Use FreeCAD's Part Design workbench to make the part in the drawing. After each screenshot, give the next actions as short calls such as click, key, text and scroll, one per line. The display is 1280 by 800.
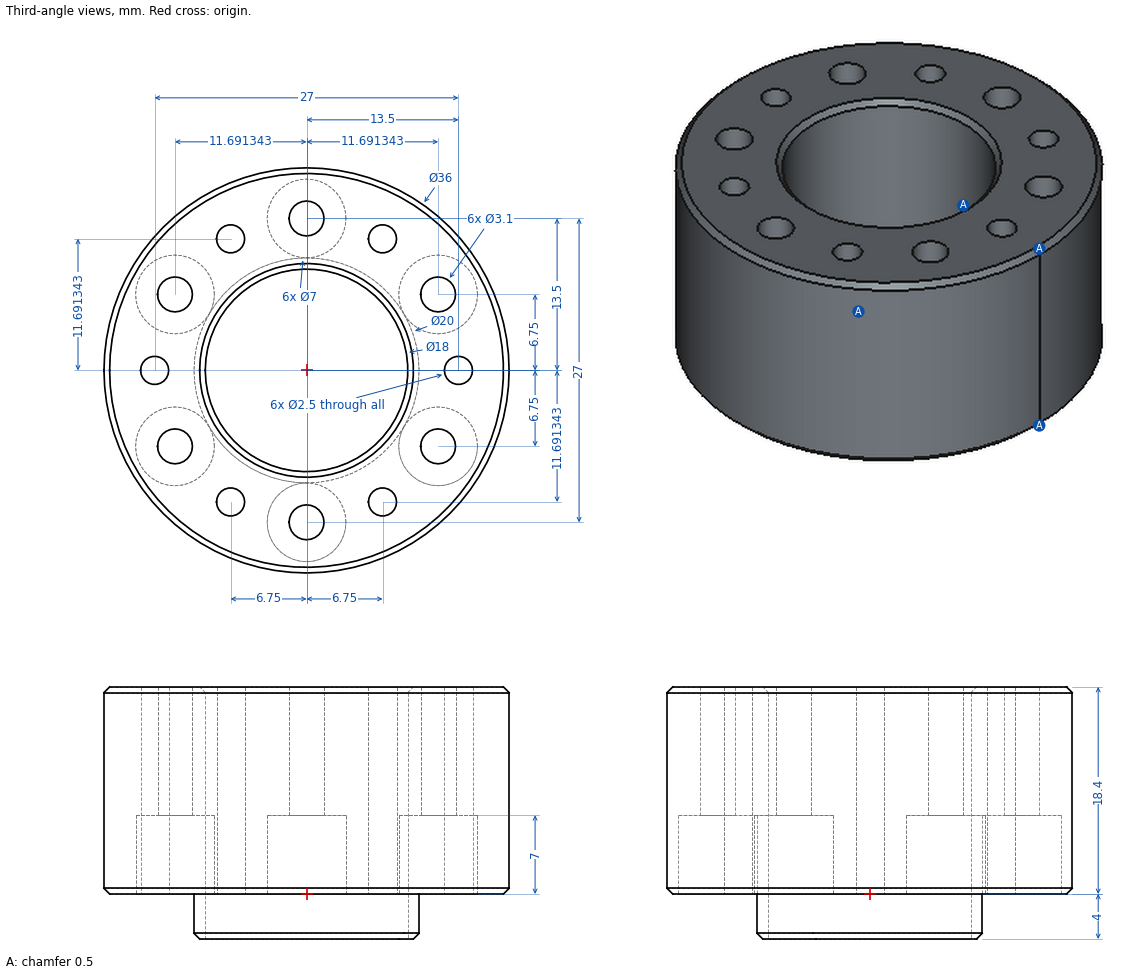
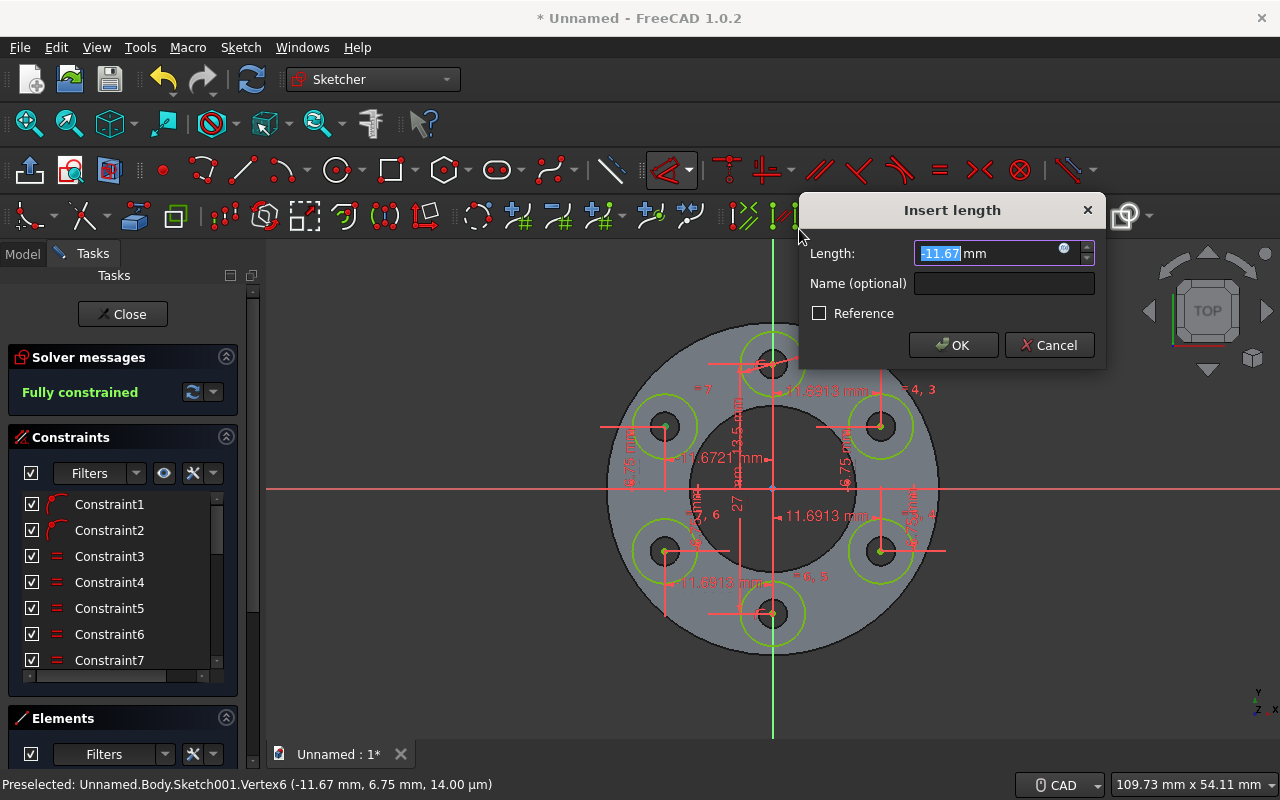
text(-11.691343)
key(Return)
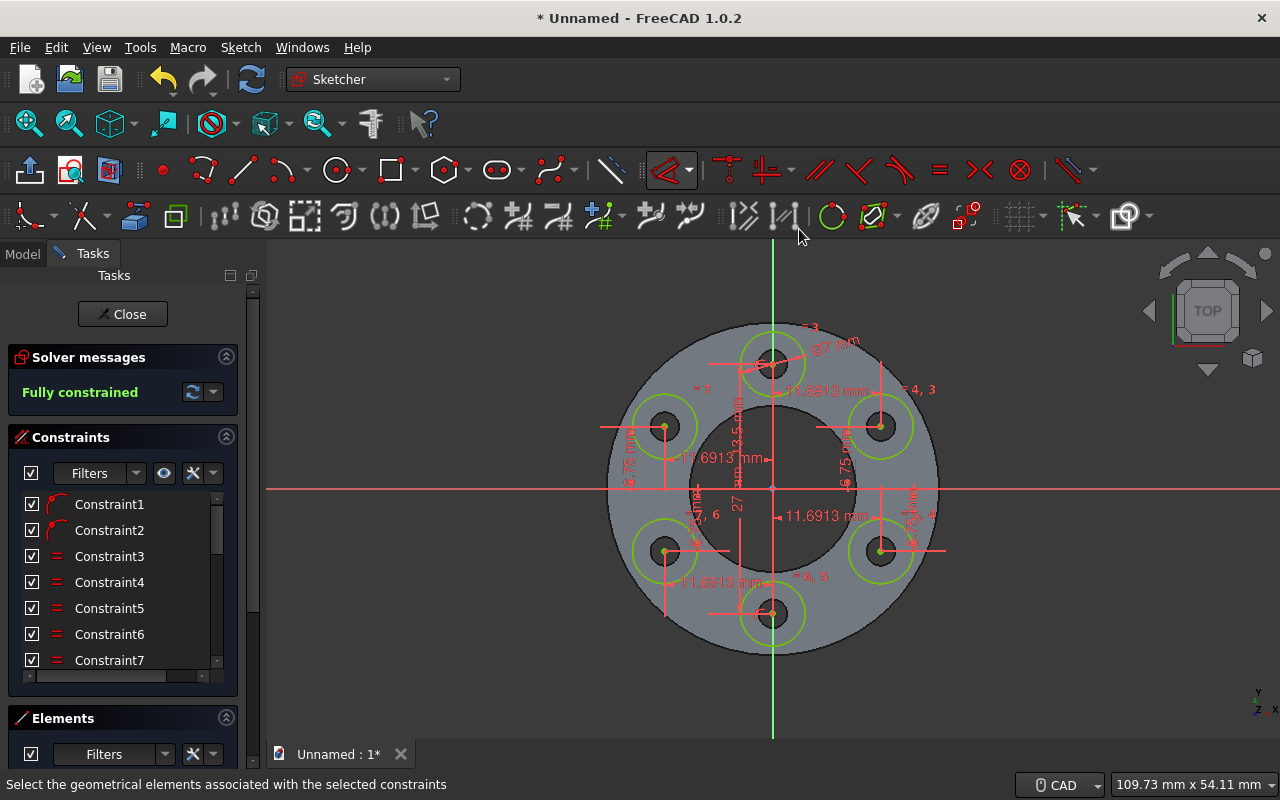
click(123, 314)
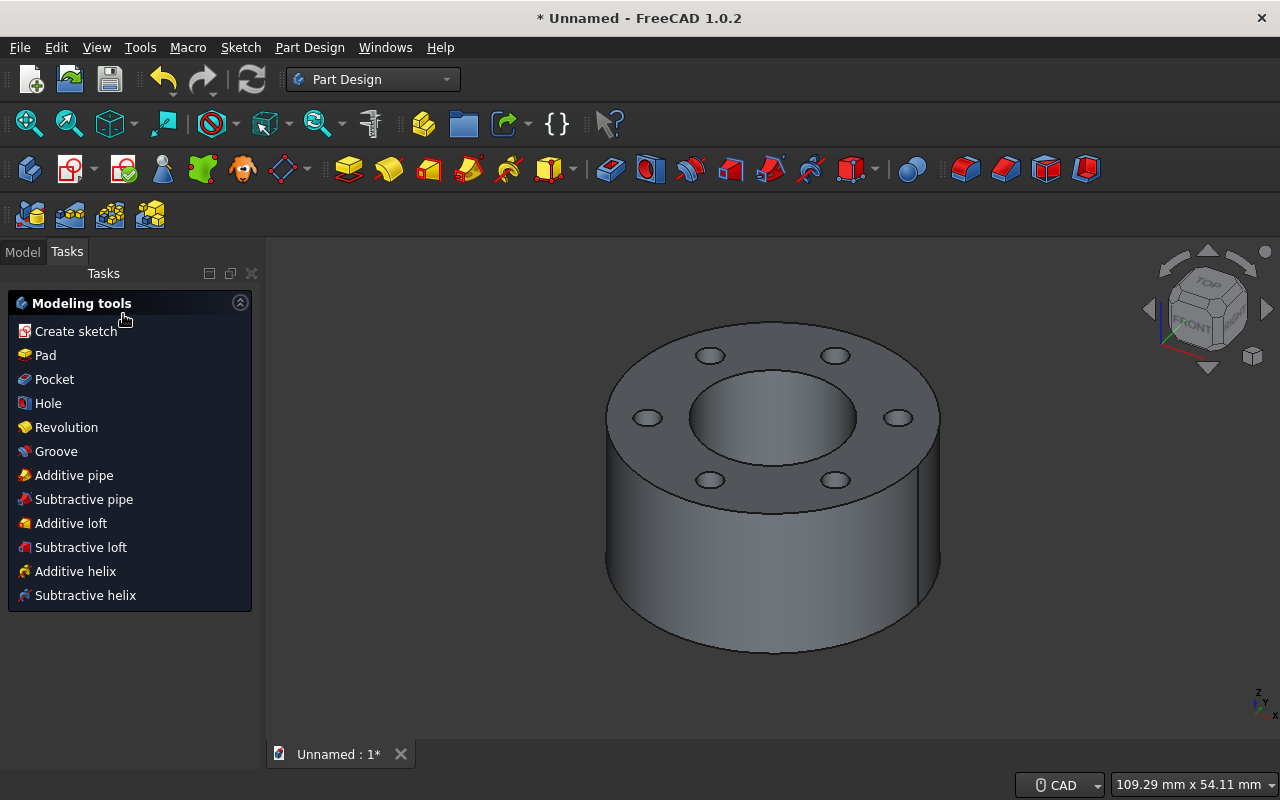
click(612, 170)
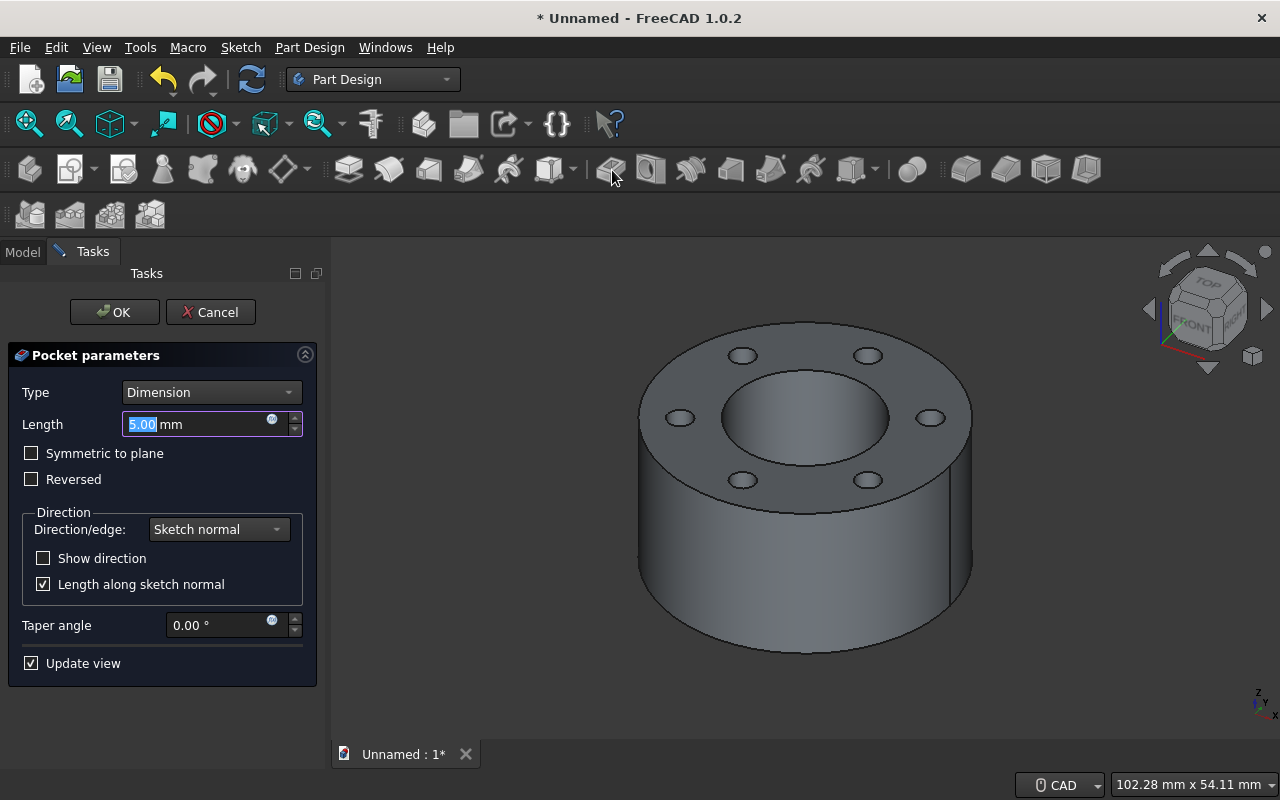
text(7)
key(Tab)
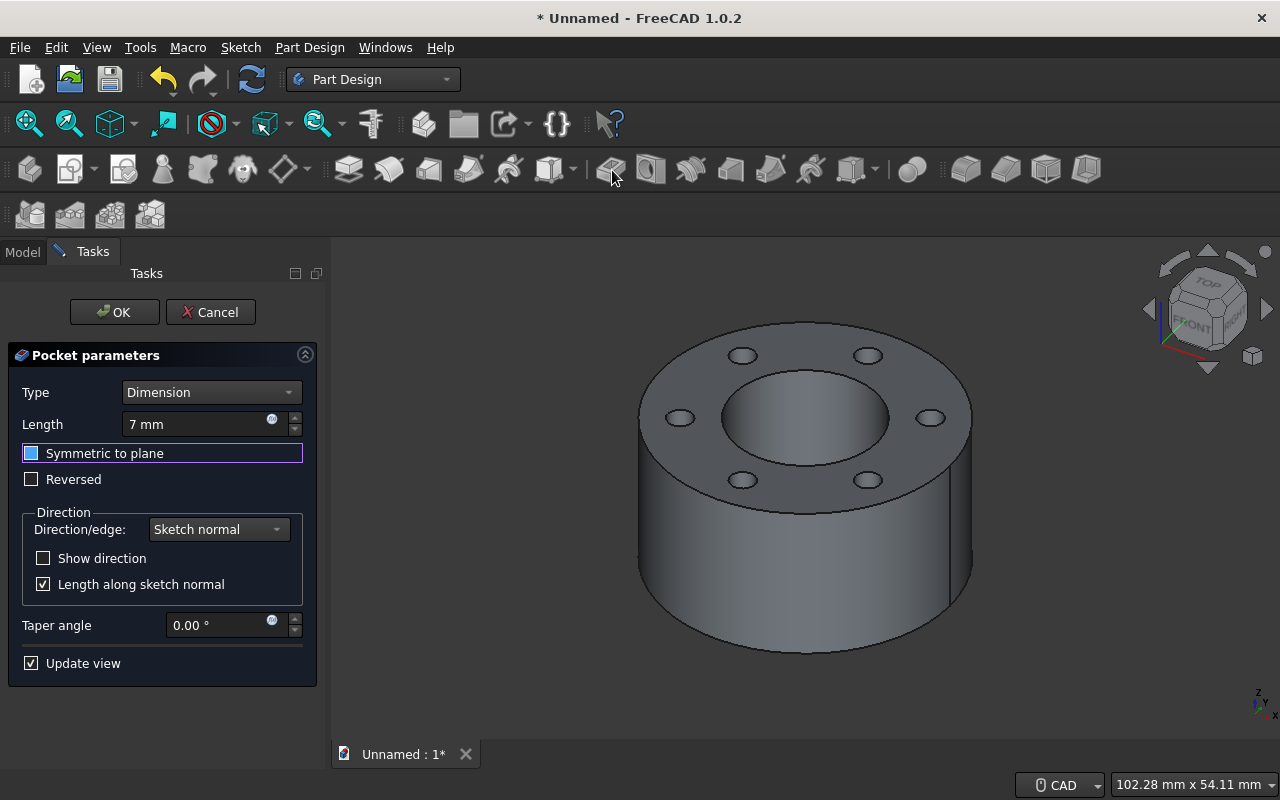
click(30, 479)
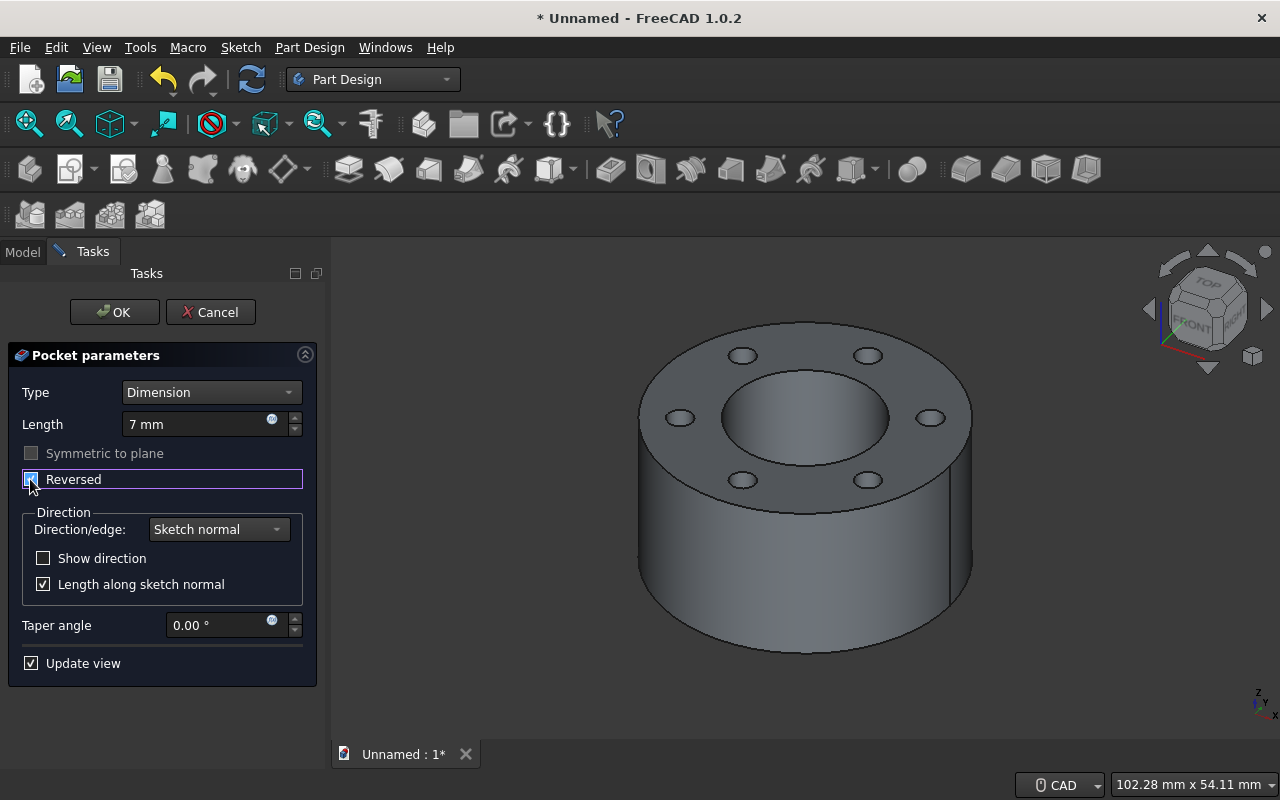
click(115, 312)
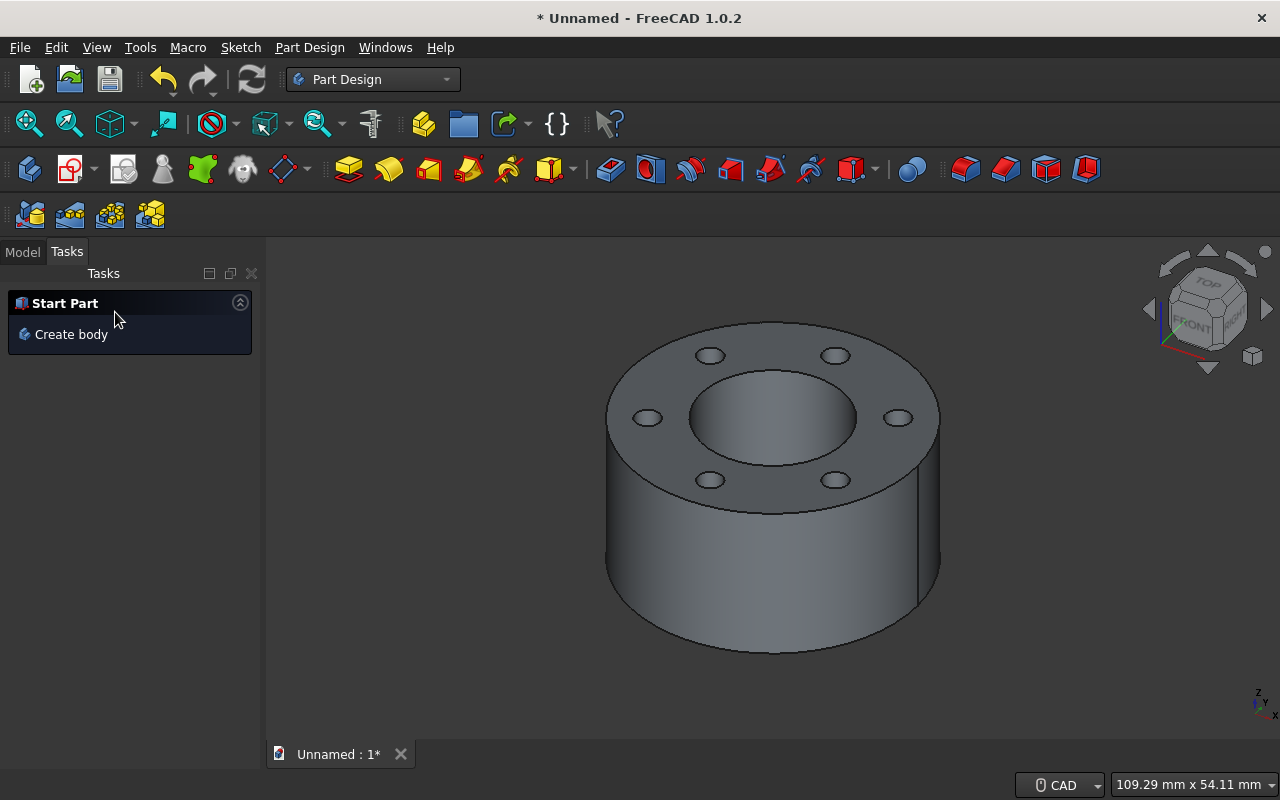
click(23, 251)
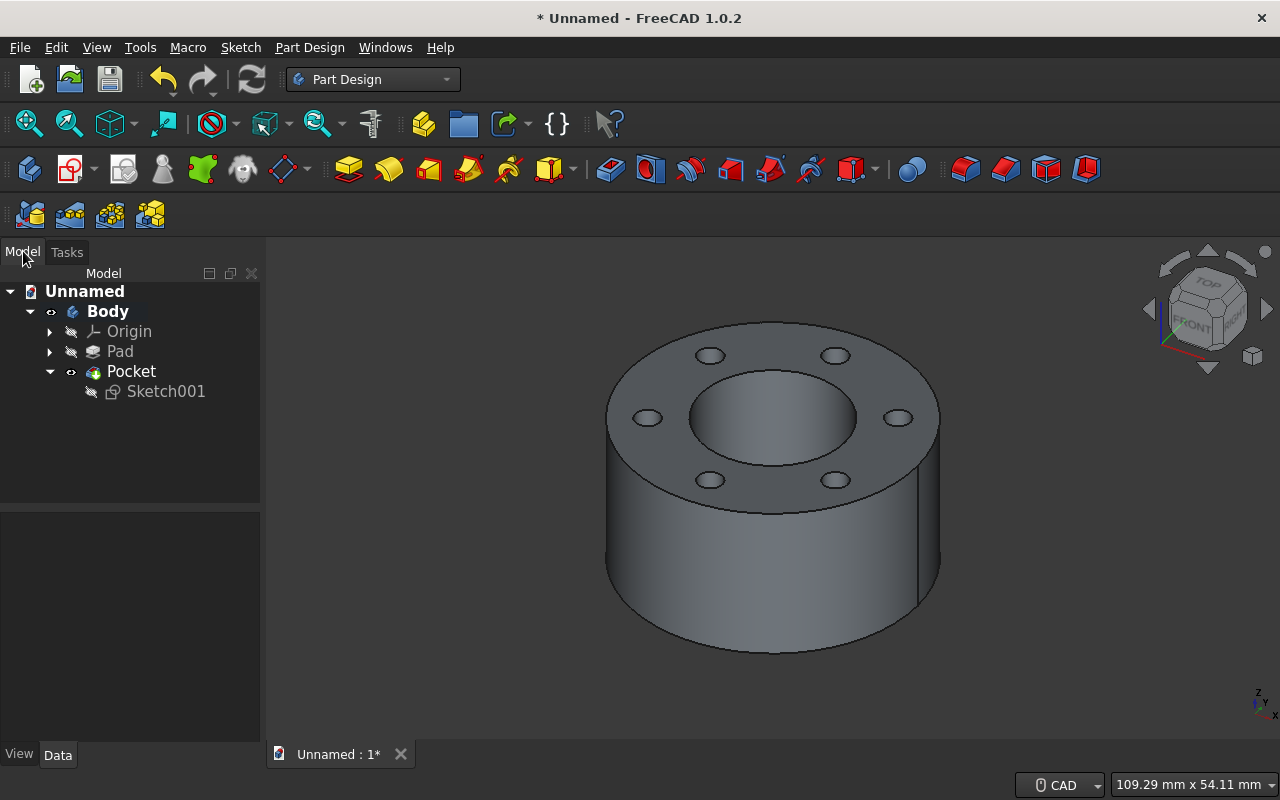
click(50, 332)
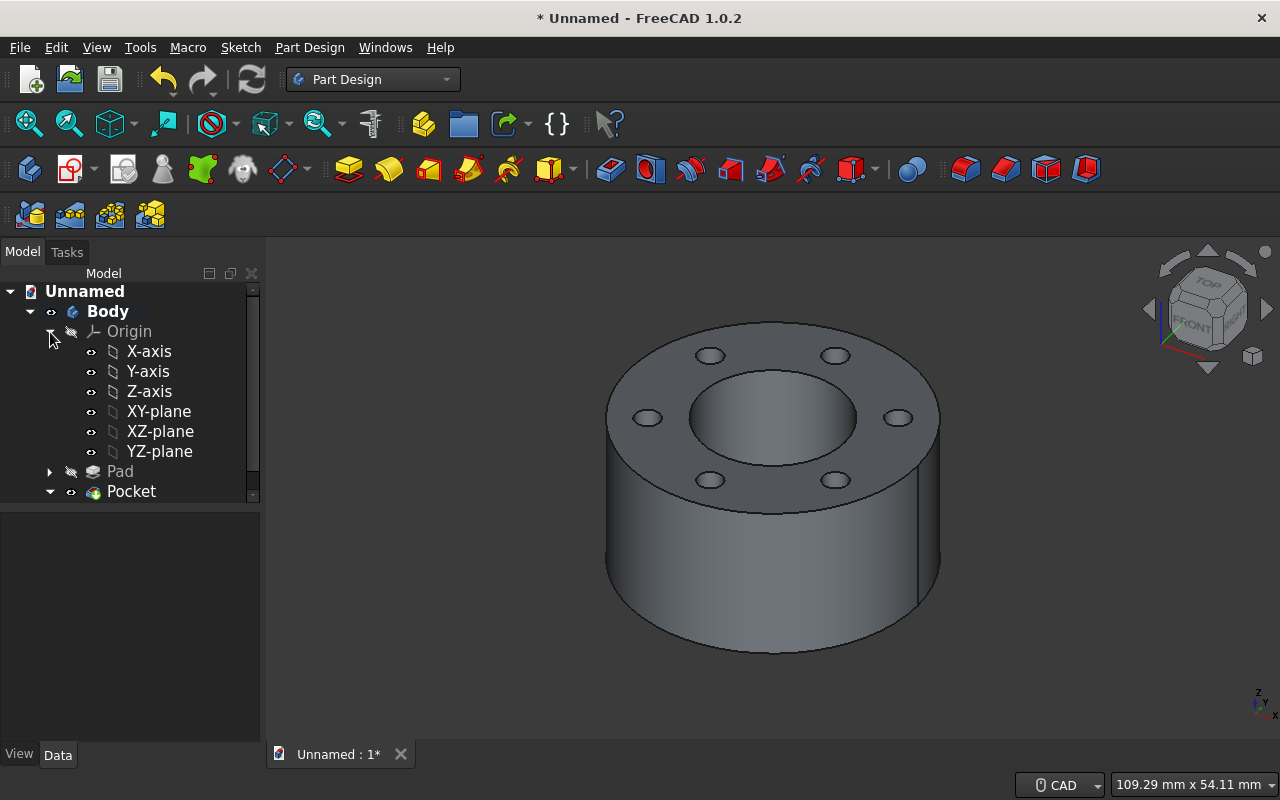
click(136, 412)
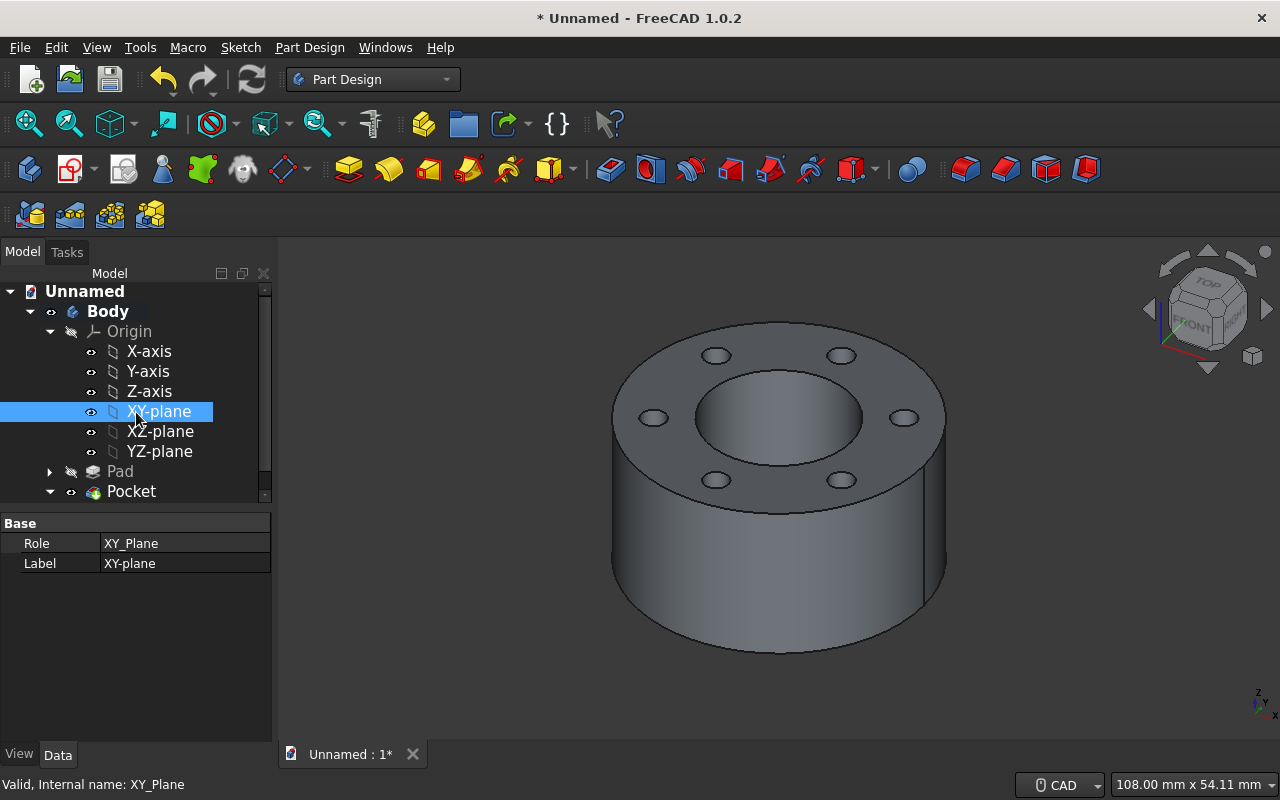
click(284, 170)